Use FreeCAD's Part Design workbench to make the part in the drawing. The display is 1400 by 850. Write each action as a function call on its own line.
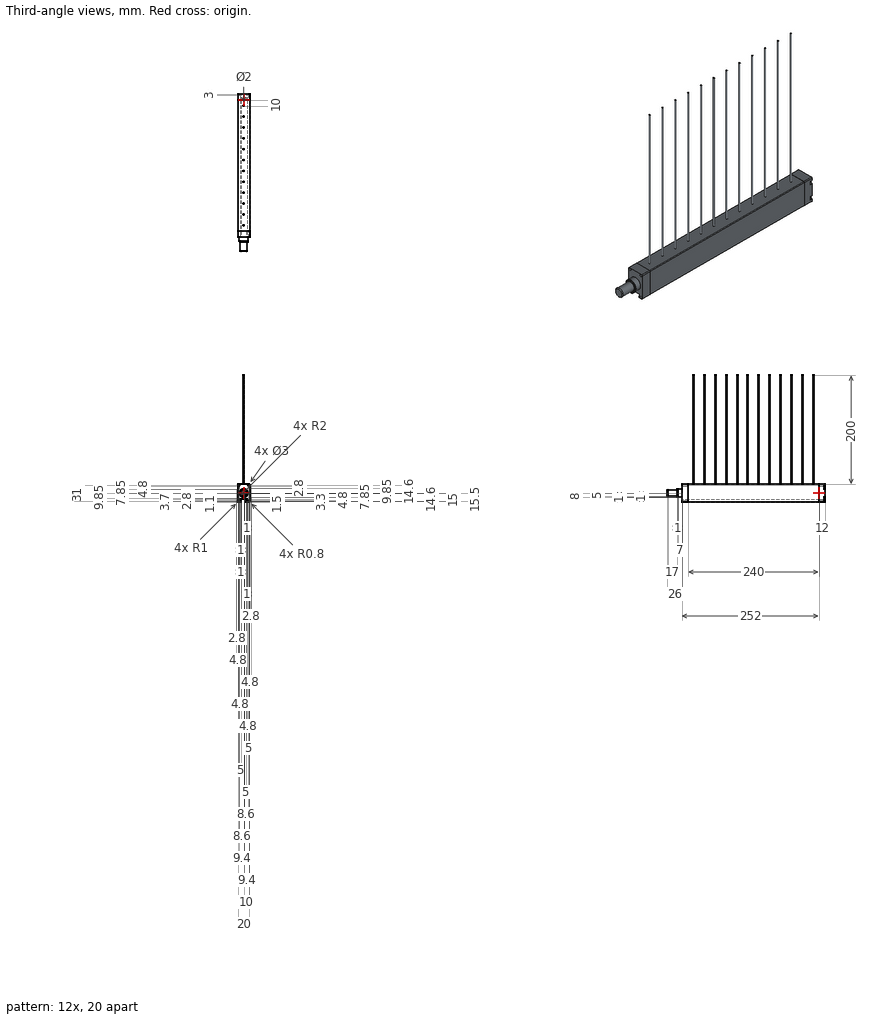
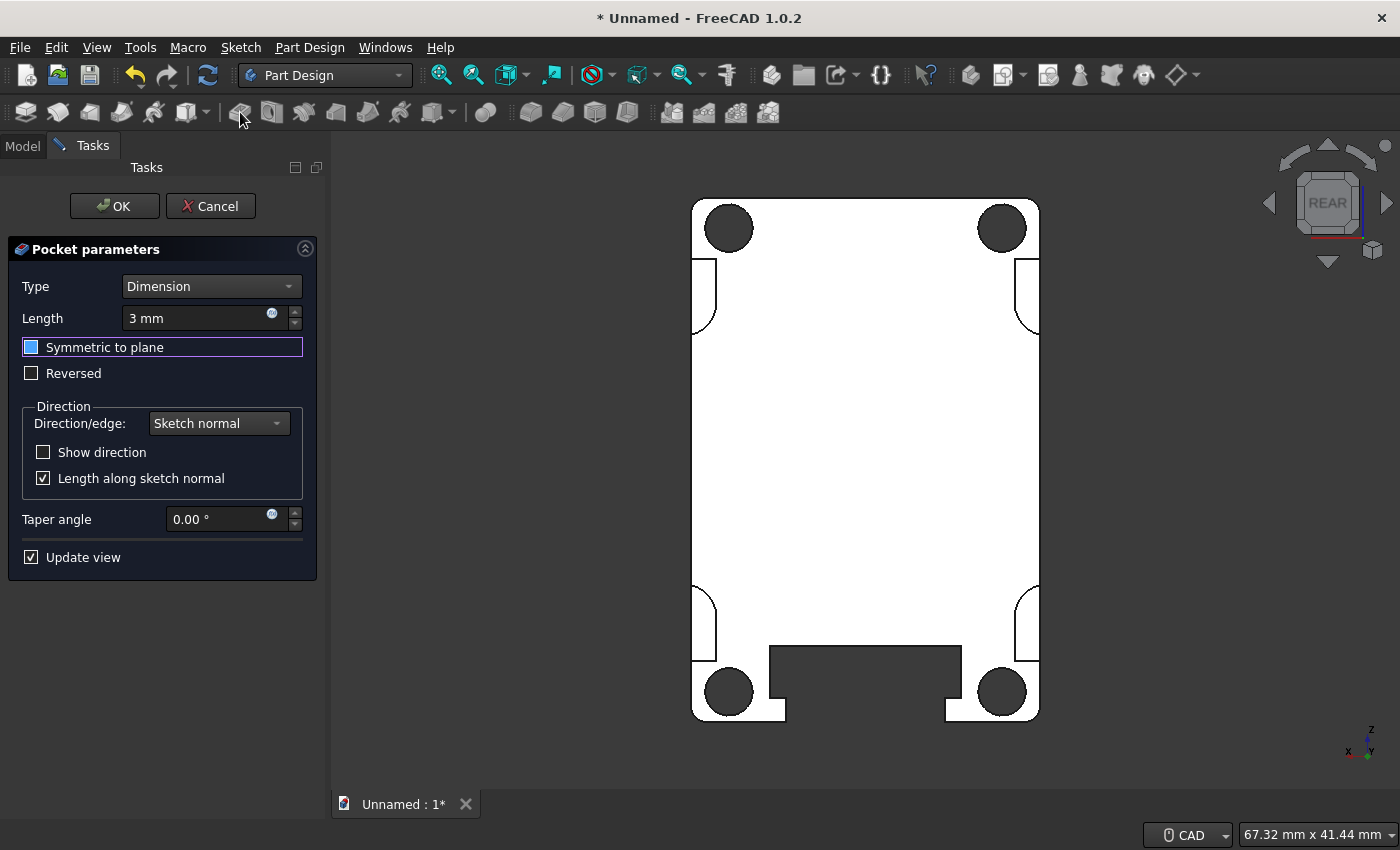
click(115, 206)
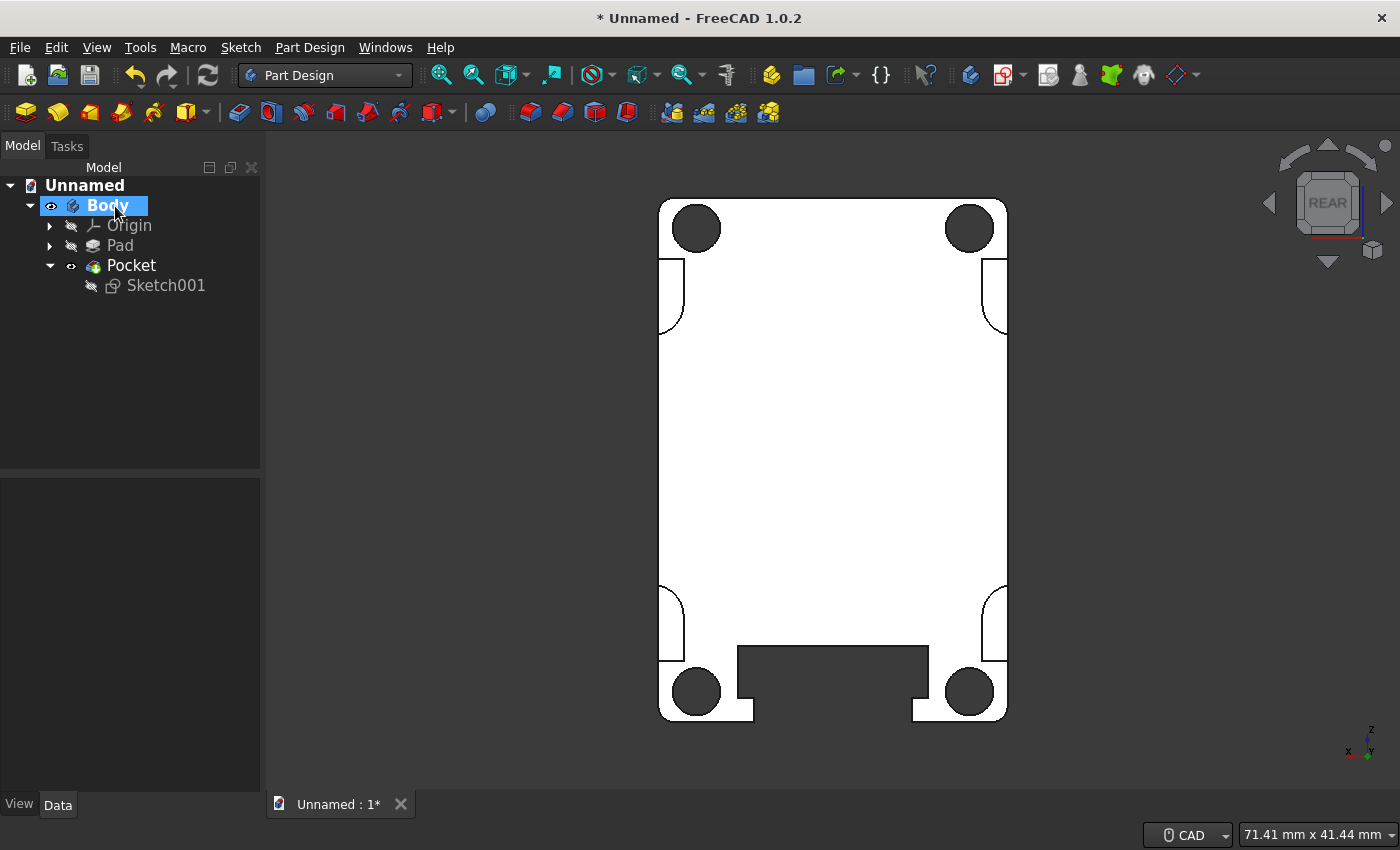
click(1004, 76)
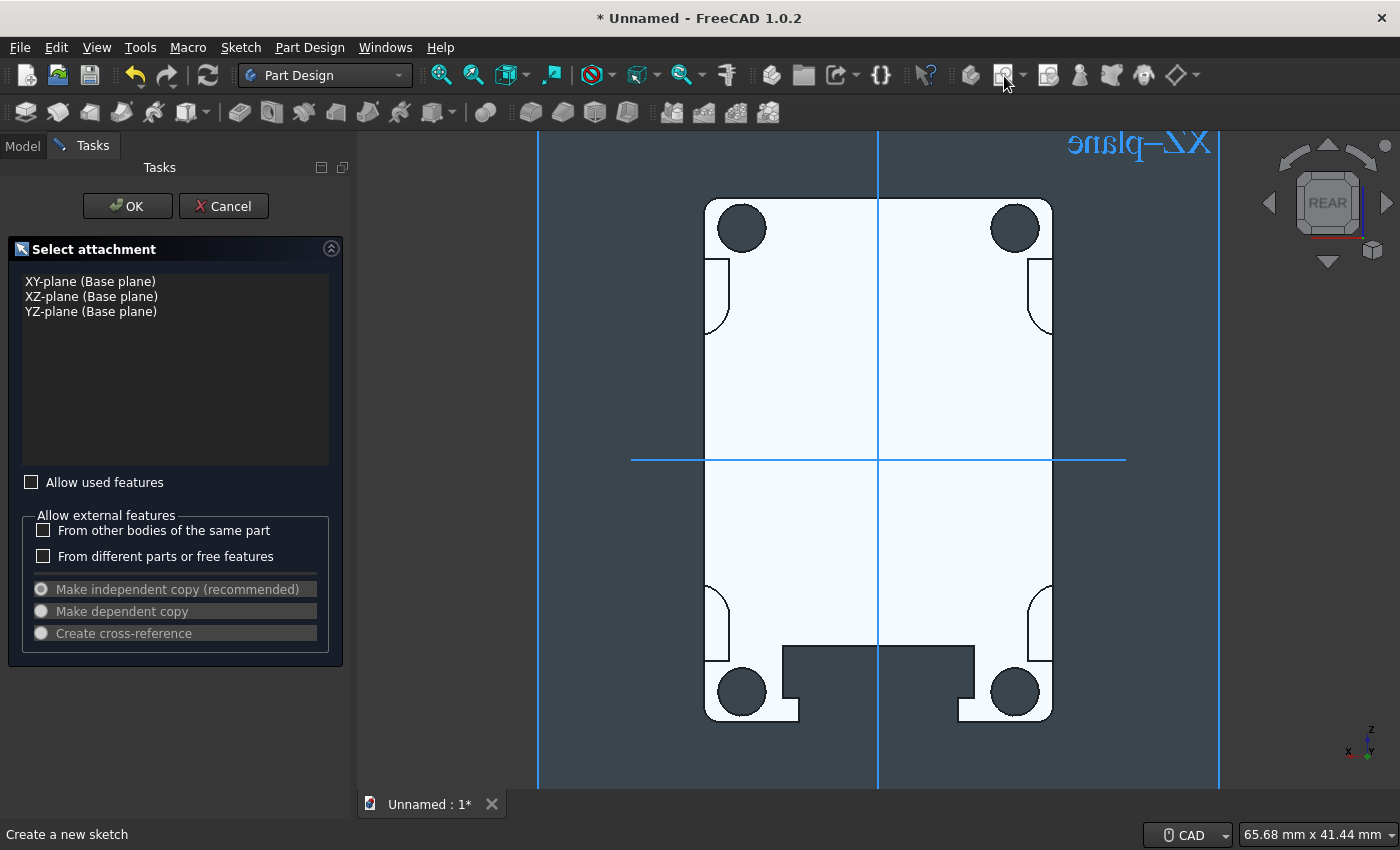
click(82, 296)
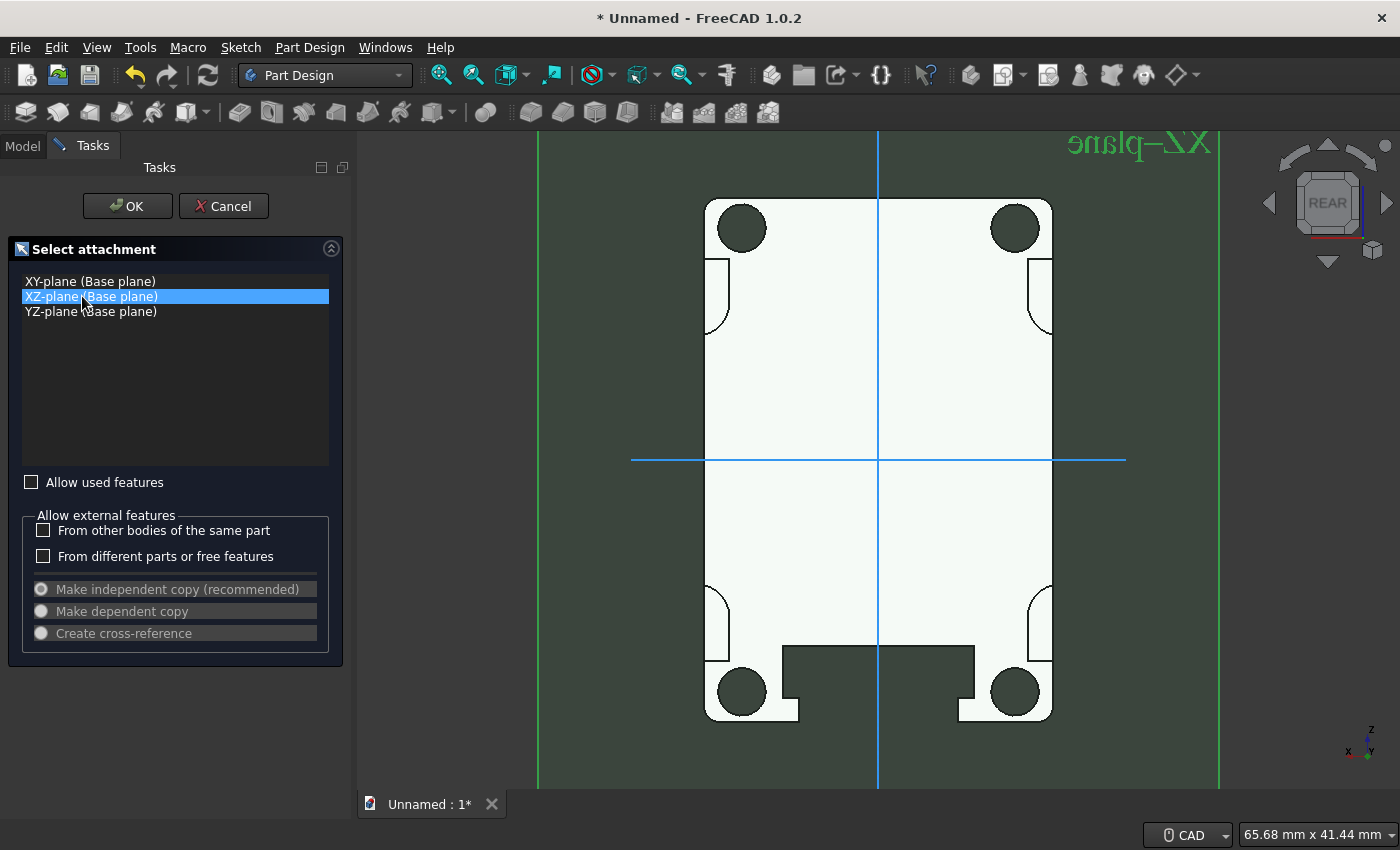
click(128, 206)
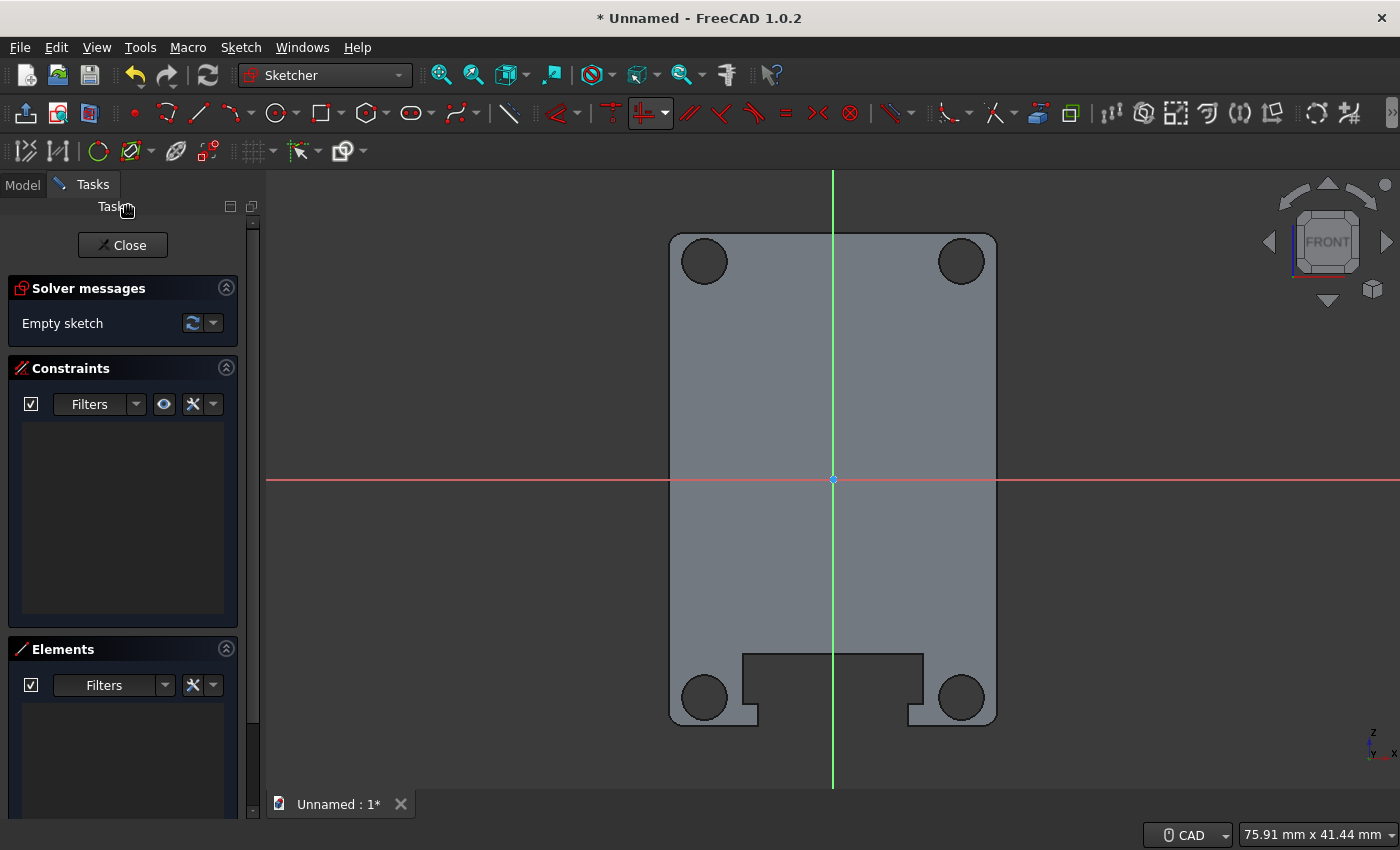
click(200, 114)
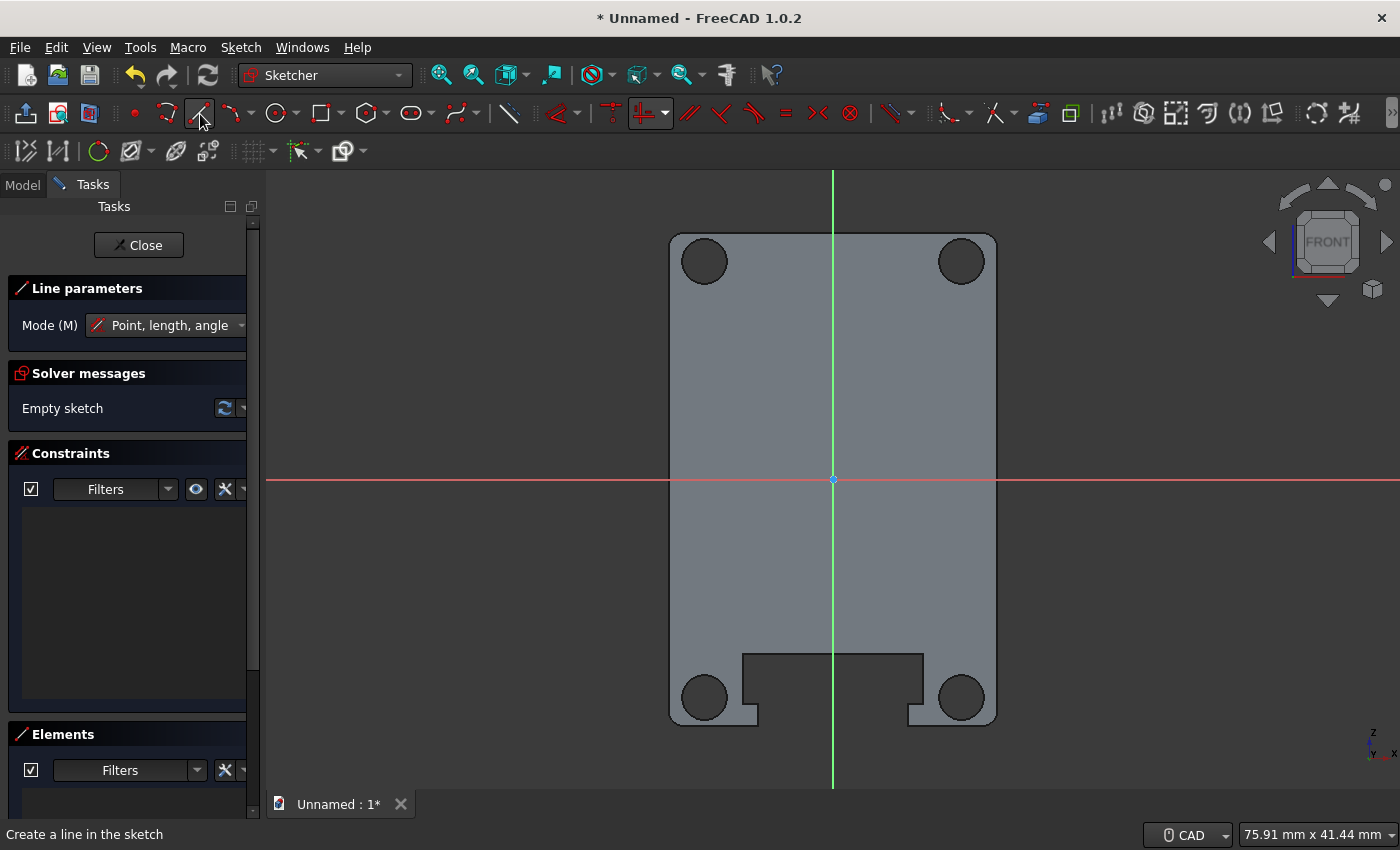
click(994, 711)
click(994, 248)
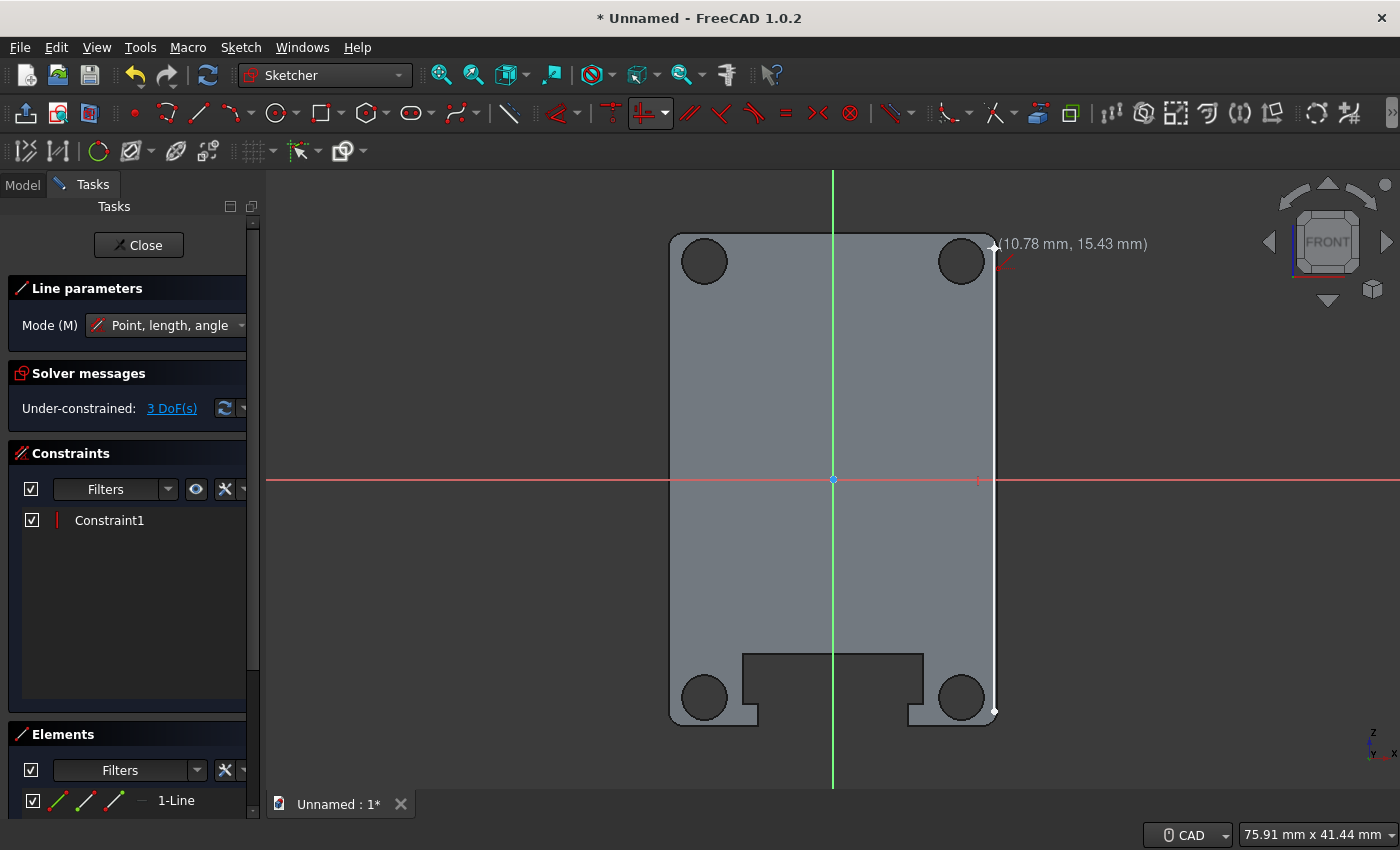
click(982, 236)
click(684, 236)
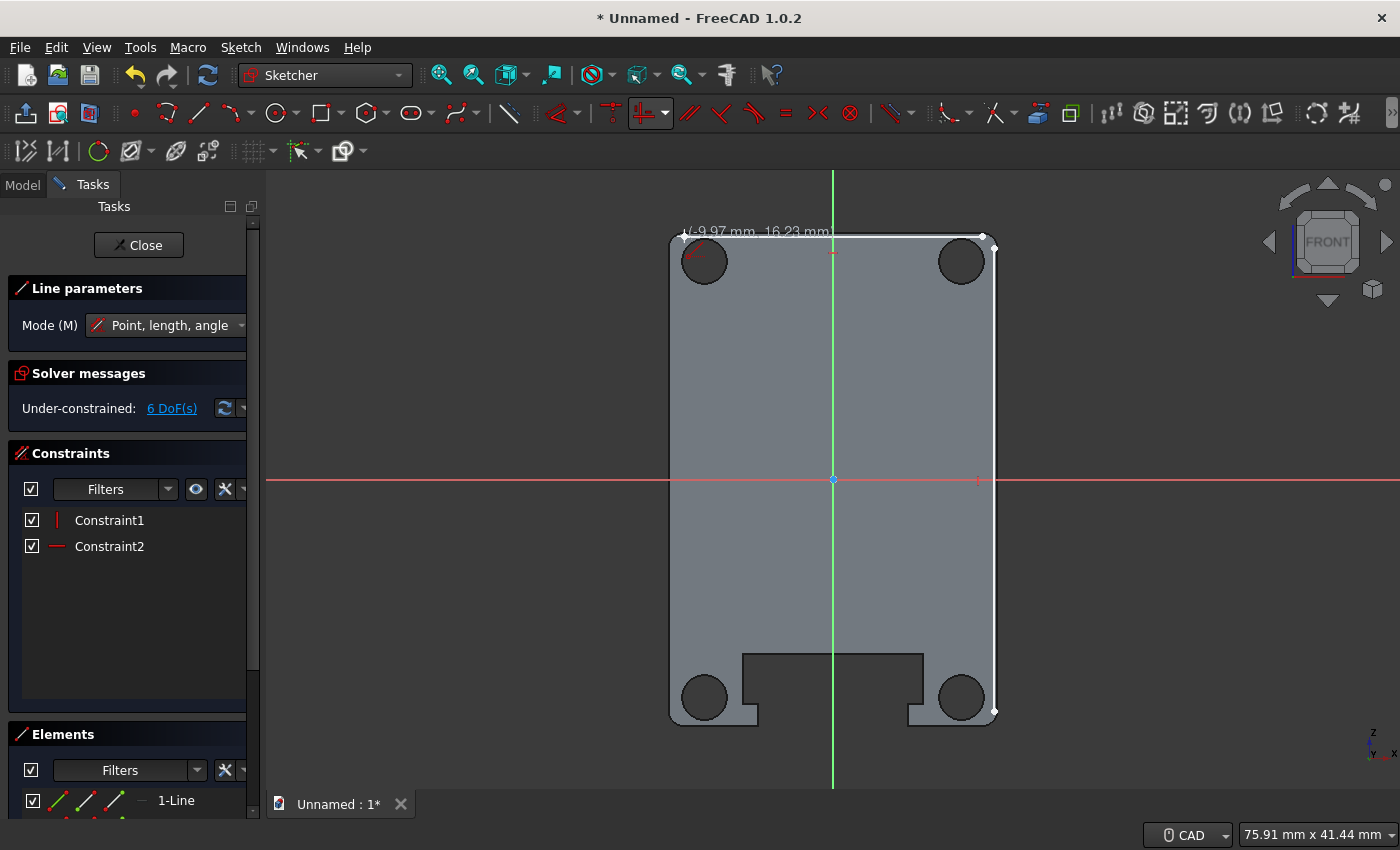
click(672, 248)
click(672, 711)